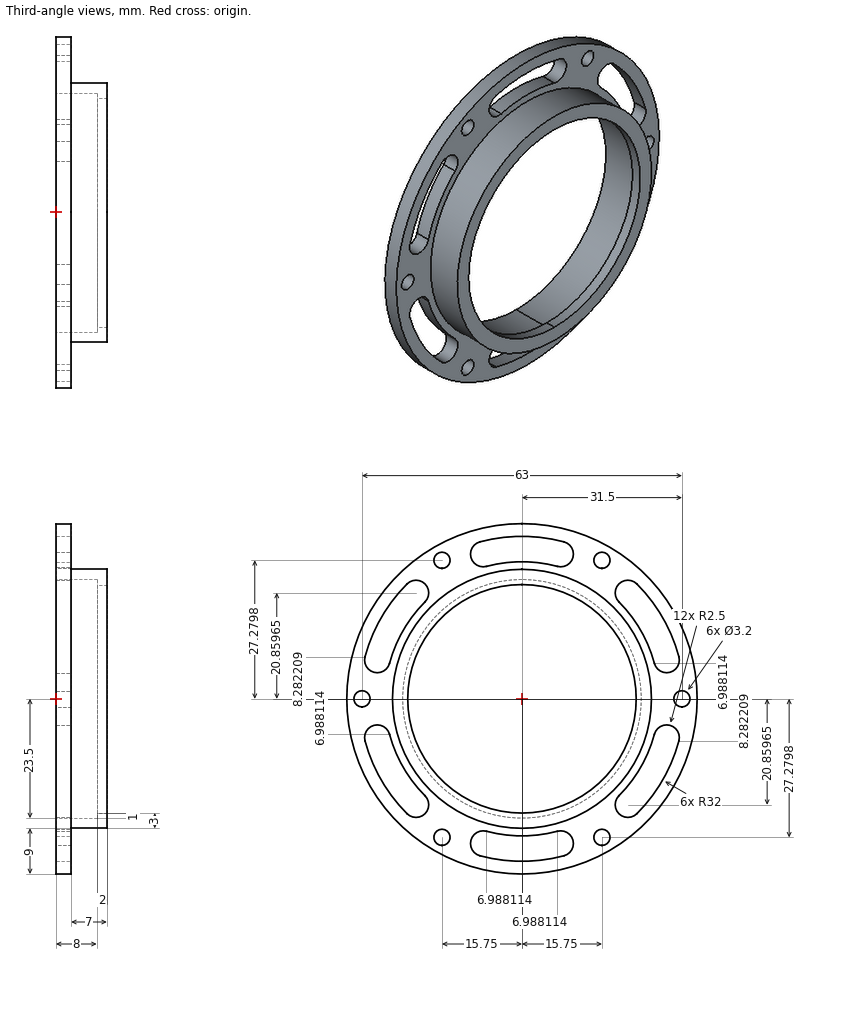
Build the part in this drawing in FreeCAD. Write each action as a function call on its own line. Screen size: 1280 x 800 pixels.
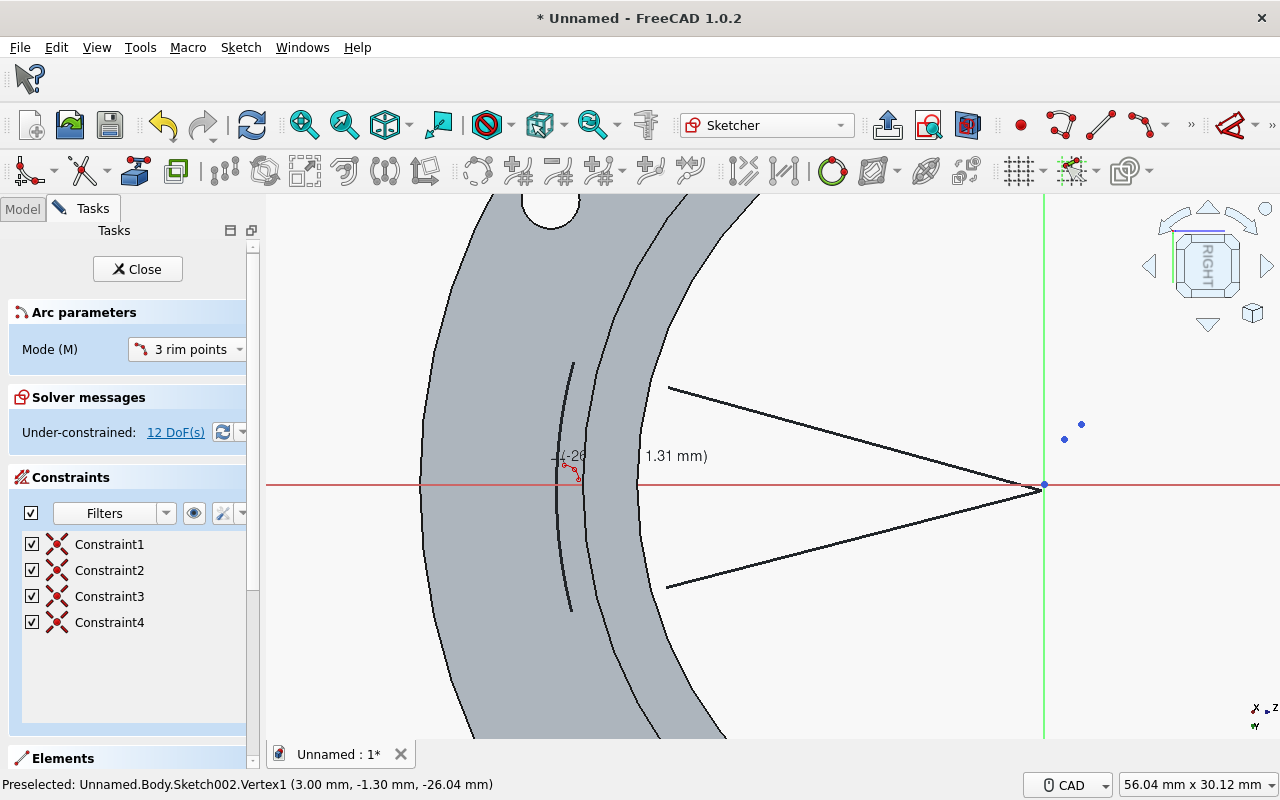
click(556, 459)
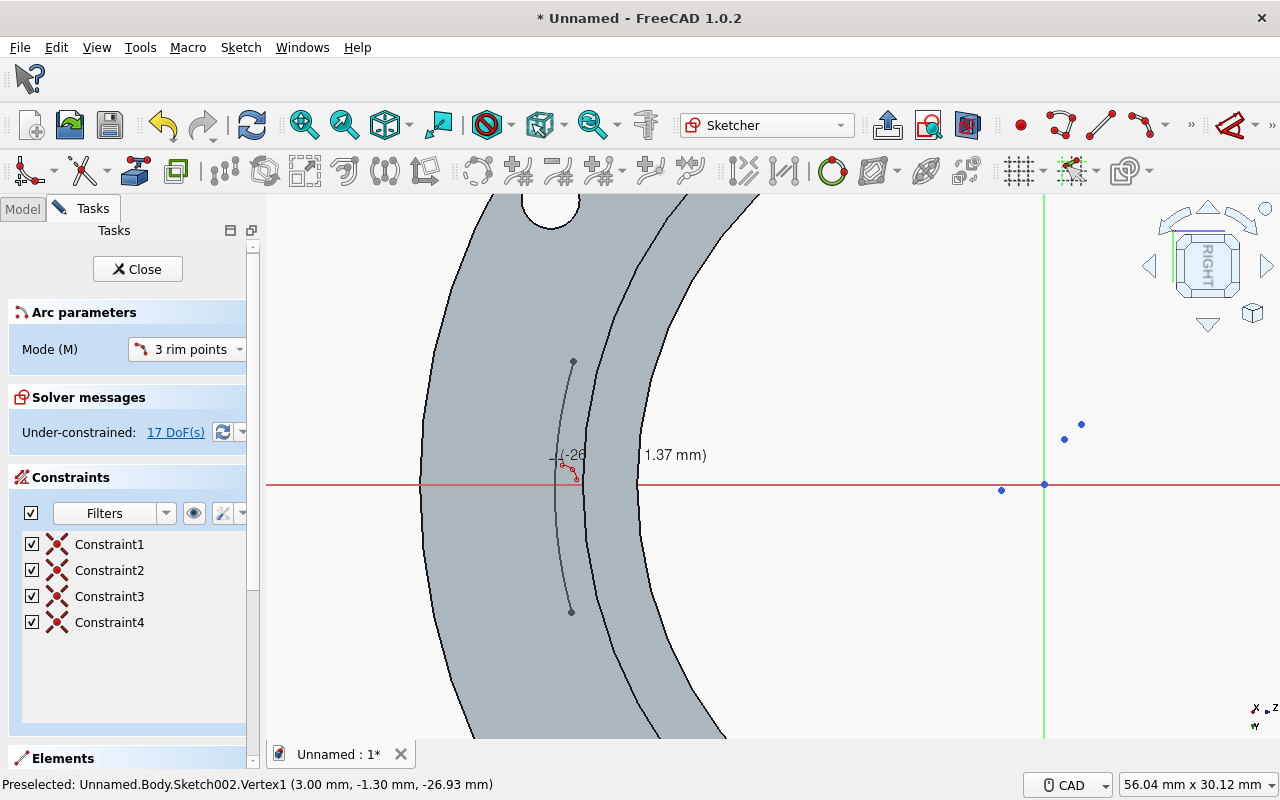
click(574, 362)
click(485, 335)
click(540, 303)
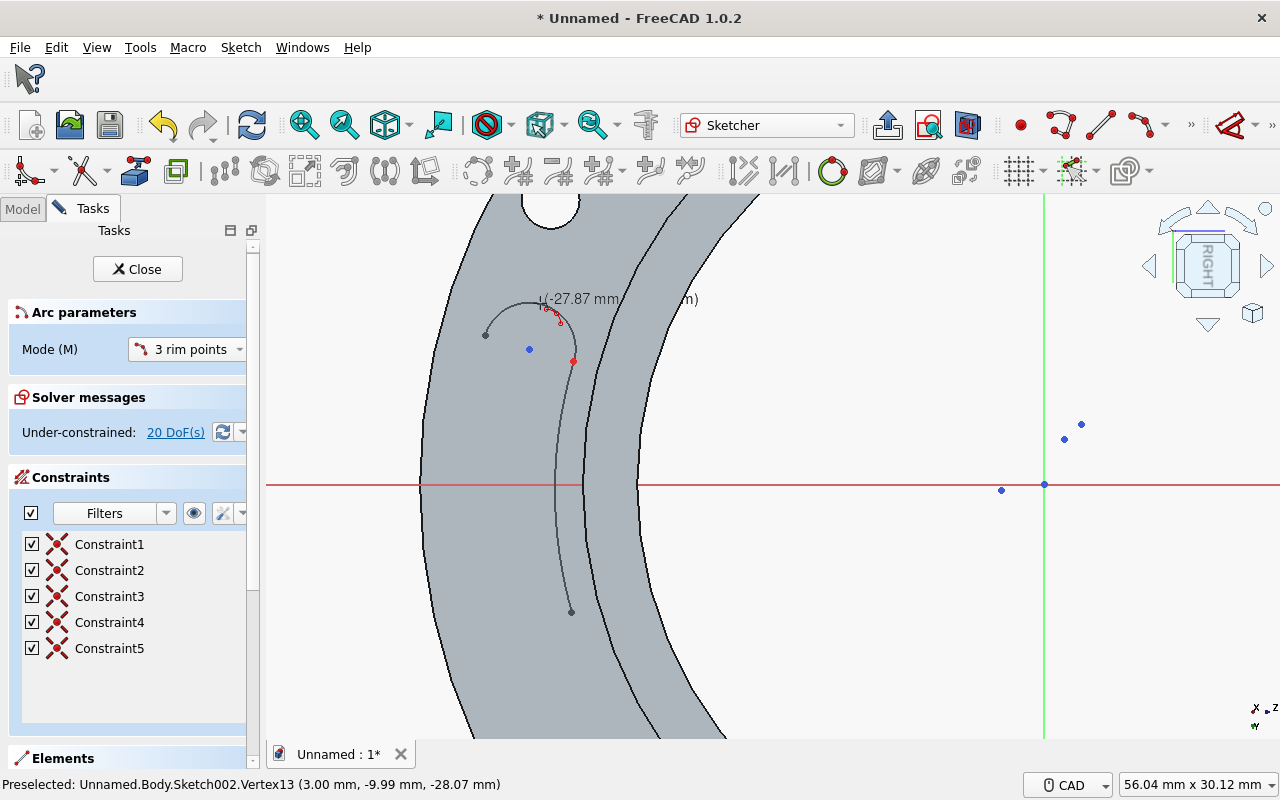
click(485, 336)
click(485, 635)
click(466, 455)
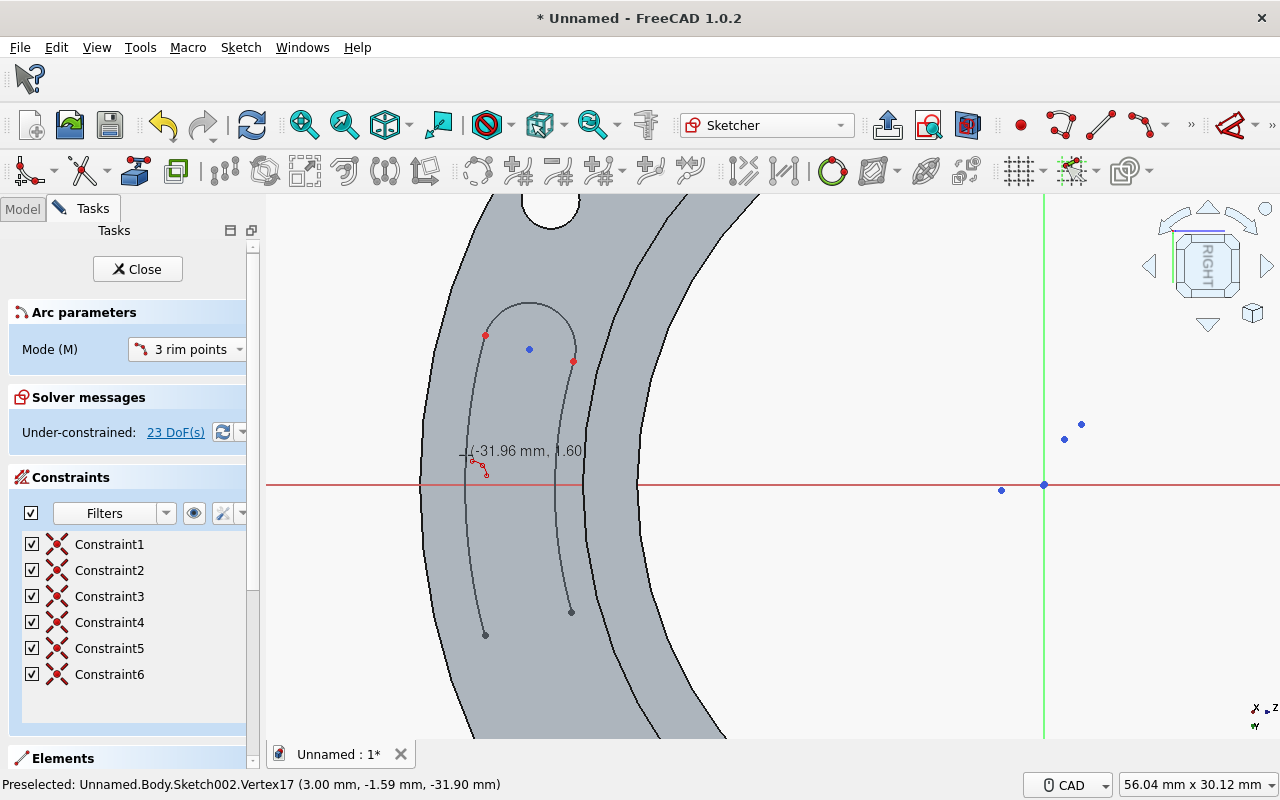
click(485, 636)
click(572, 612)
click(540, 667)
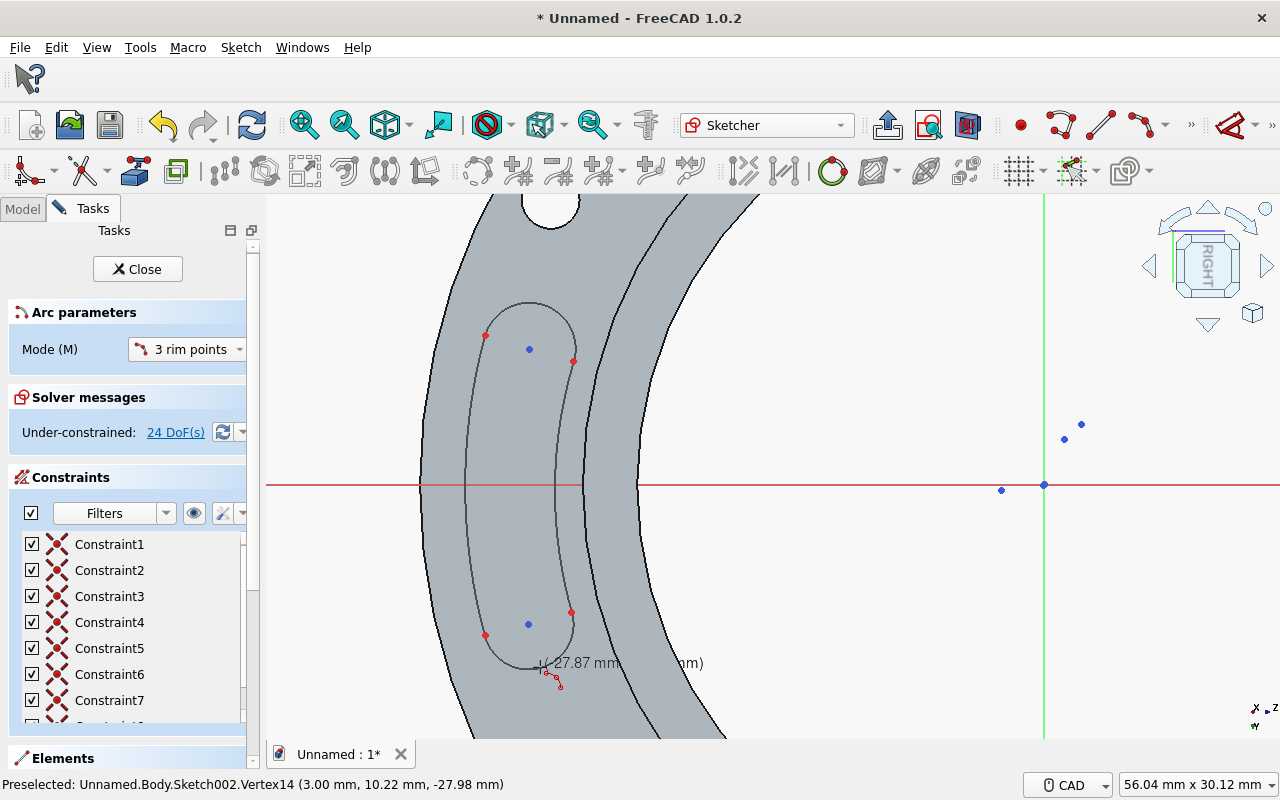
scroll(558, 459, down, 6)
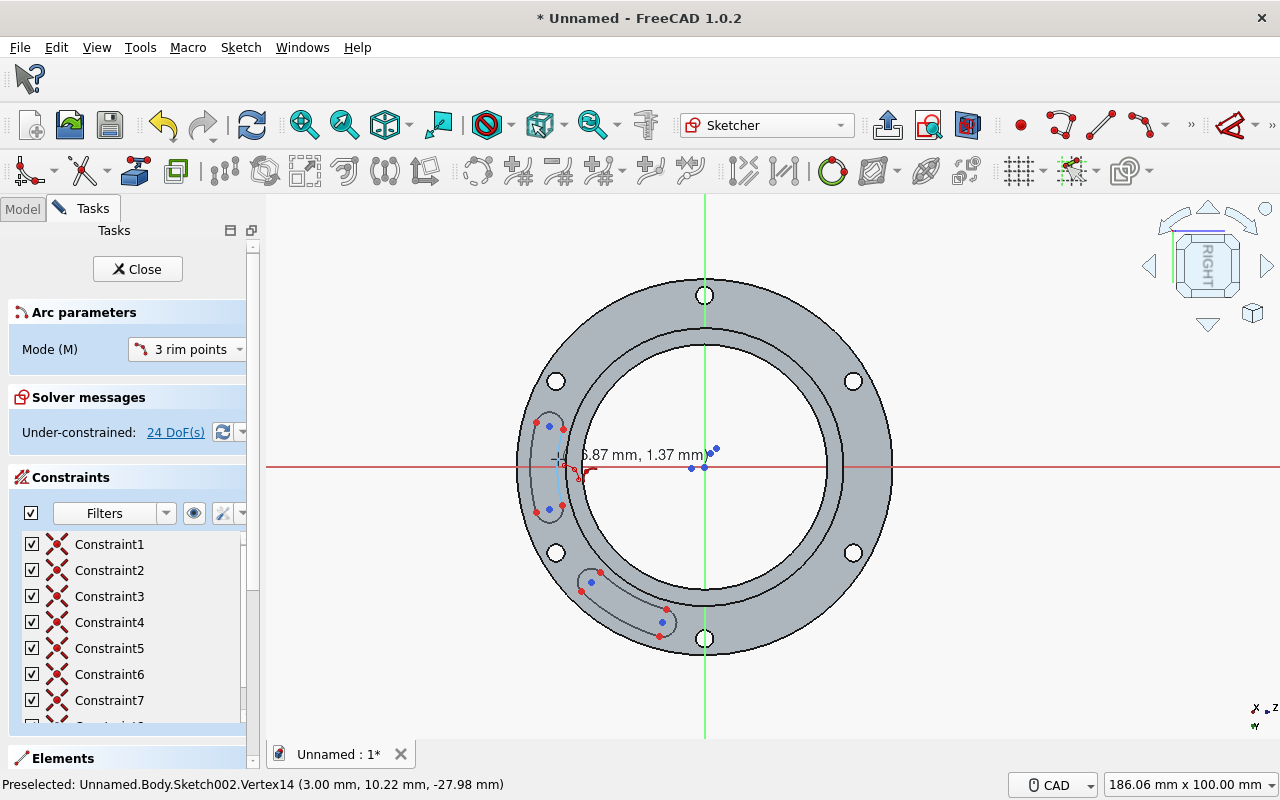
click(601, 363)
click(667, 325)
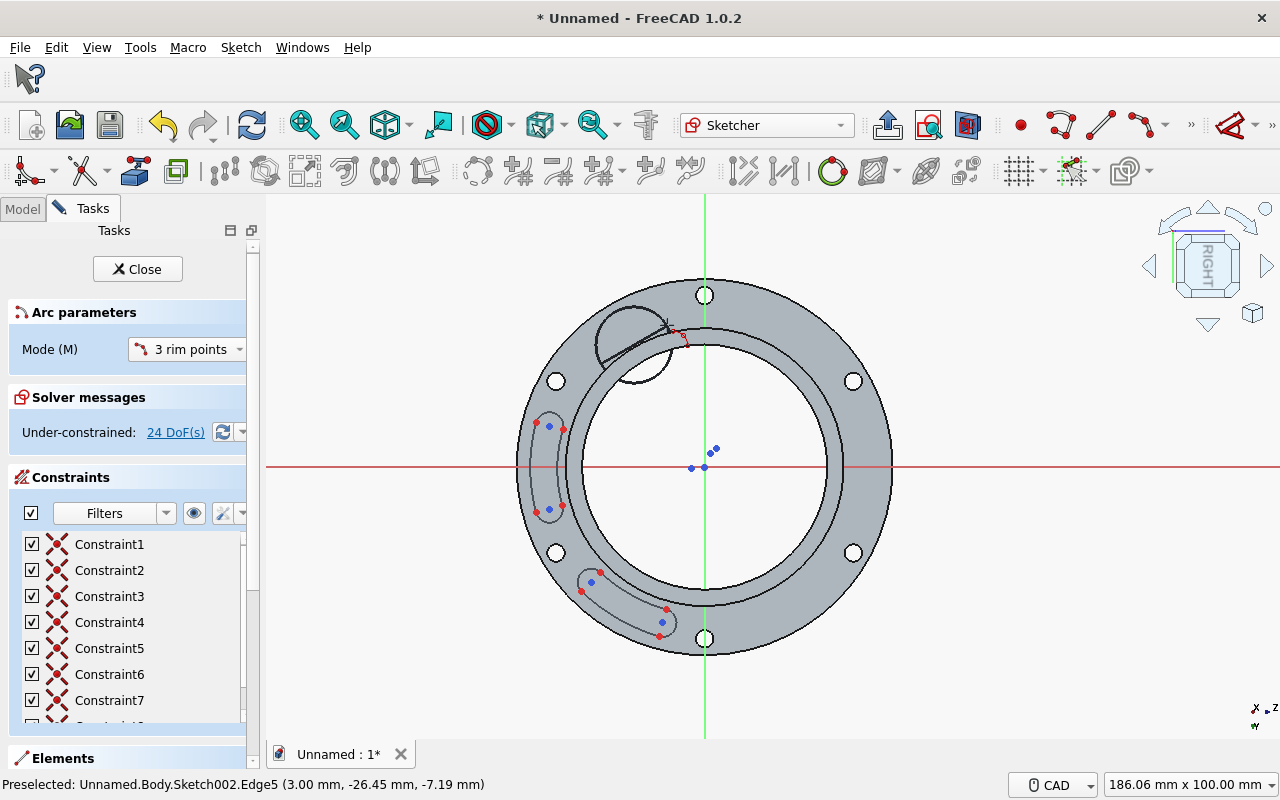
scroll(631, 340, up, 6)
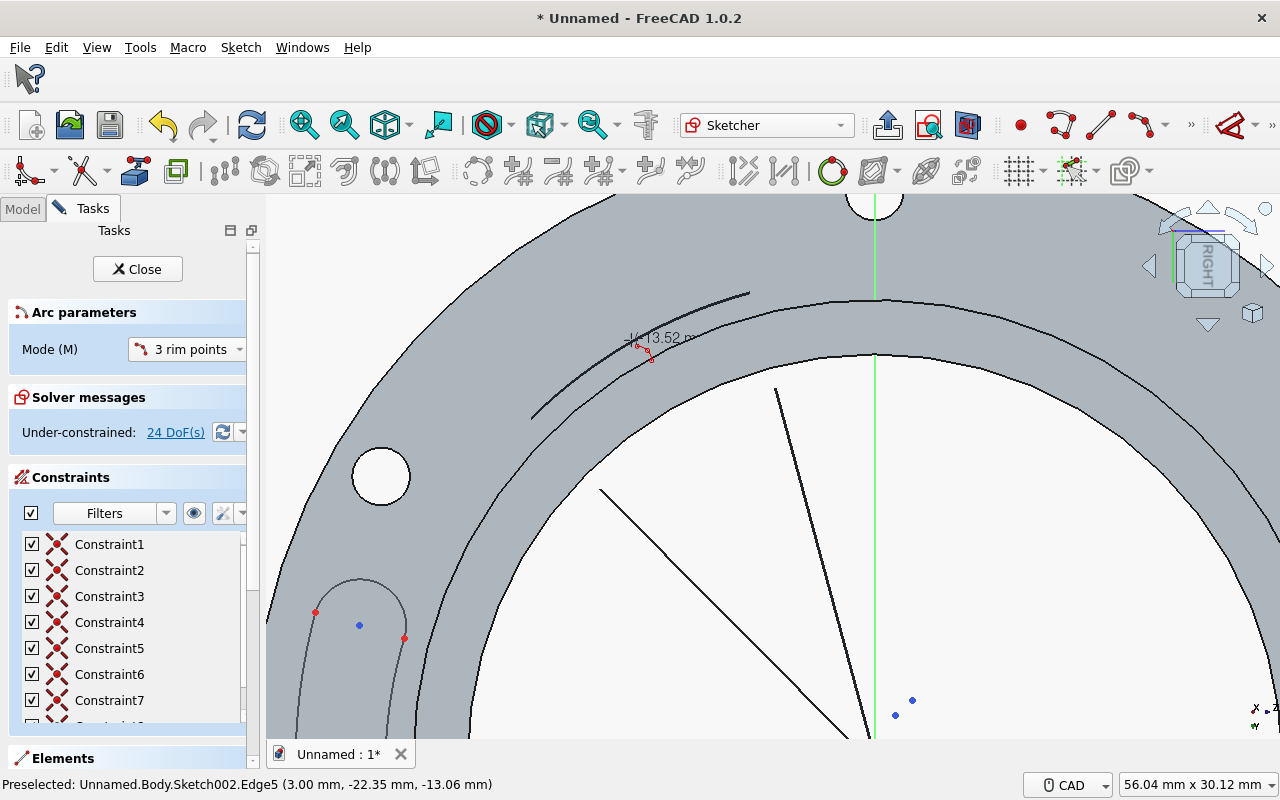
click(630, 338)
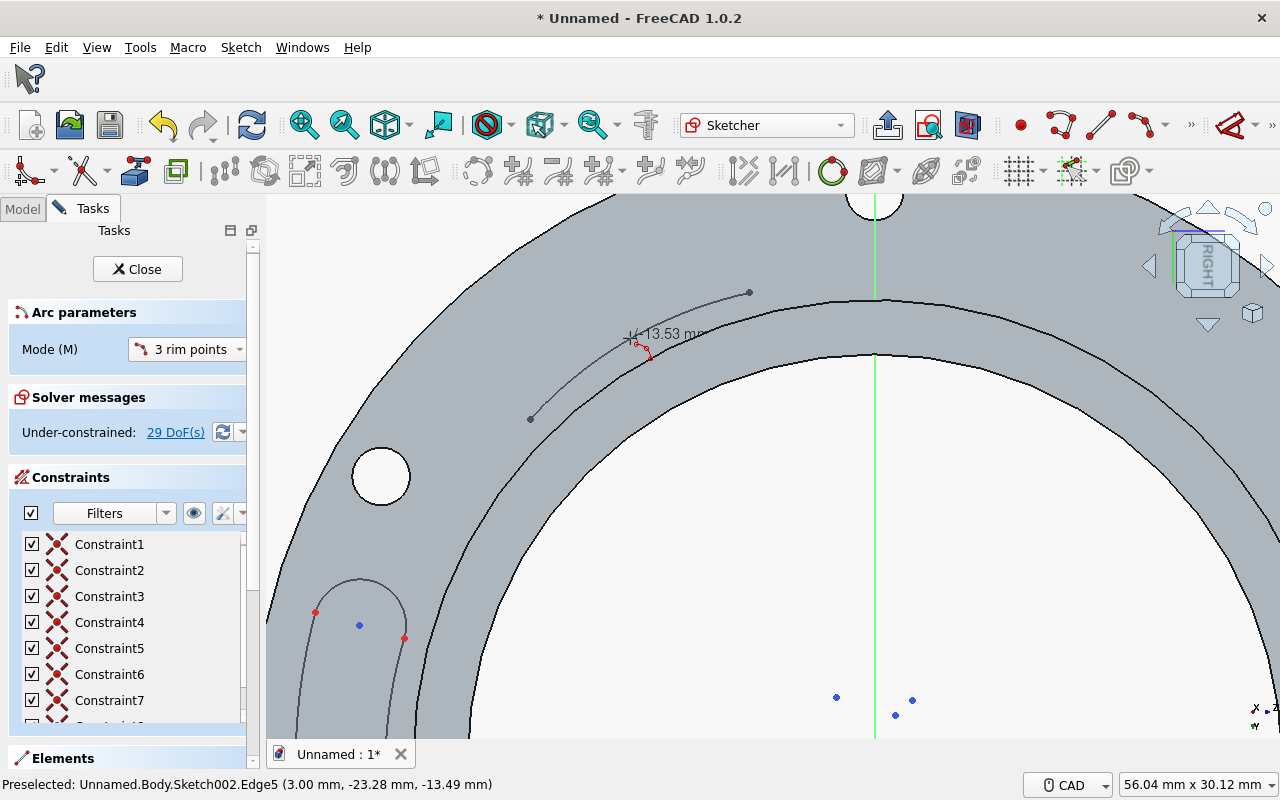
click(750, 293)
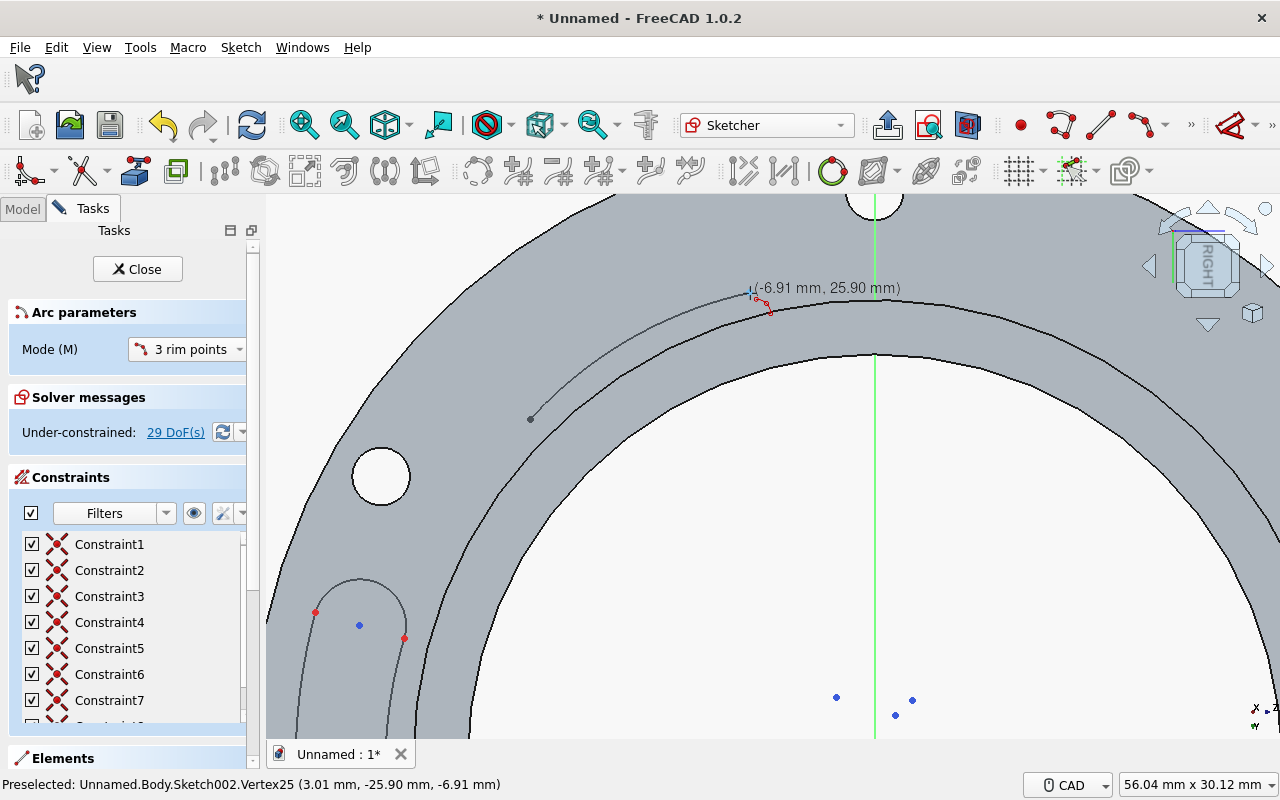
scroll(631, 339, down, 6)